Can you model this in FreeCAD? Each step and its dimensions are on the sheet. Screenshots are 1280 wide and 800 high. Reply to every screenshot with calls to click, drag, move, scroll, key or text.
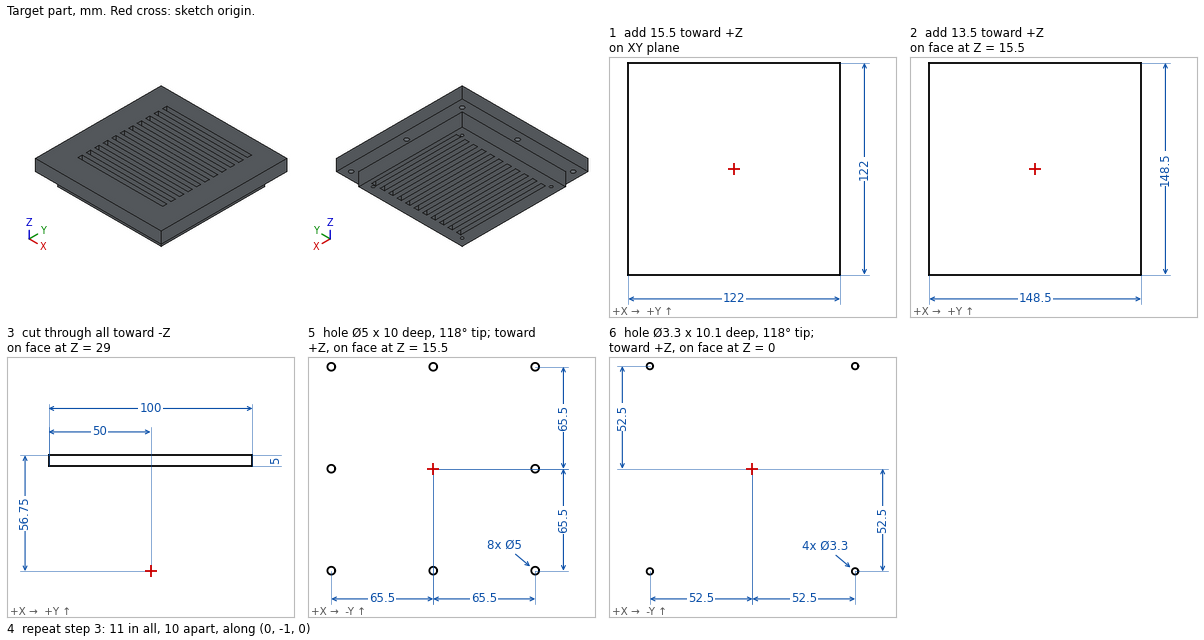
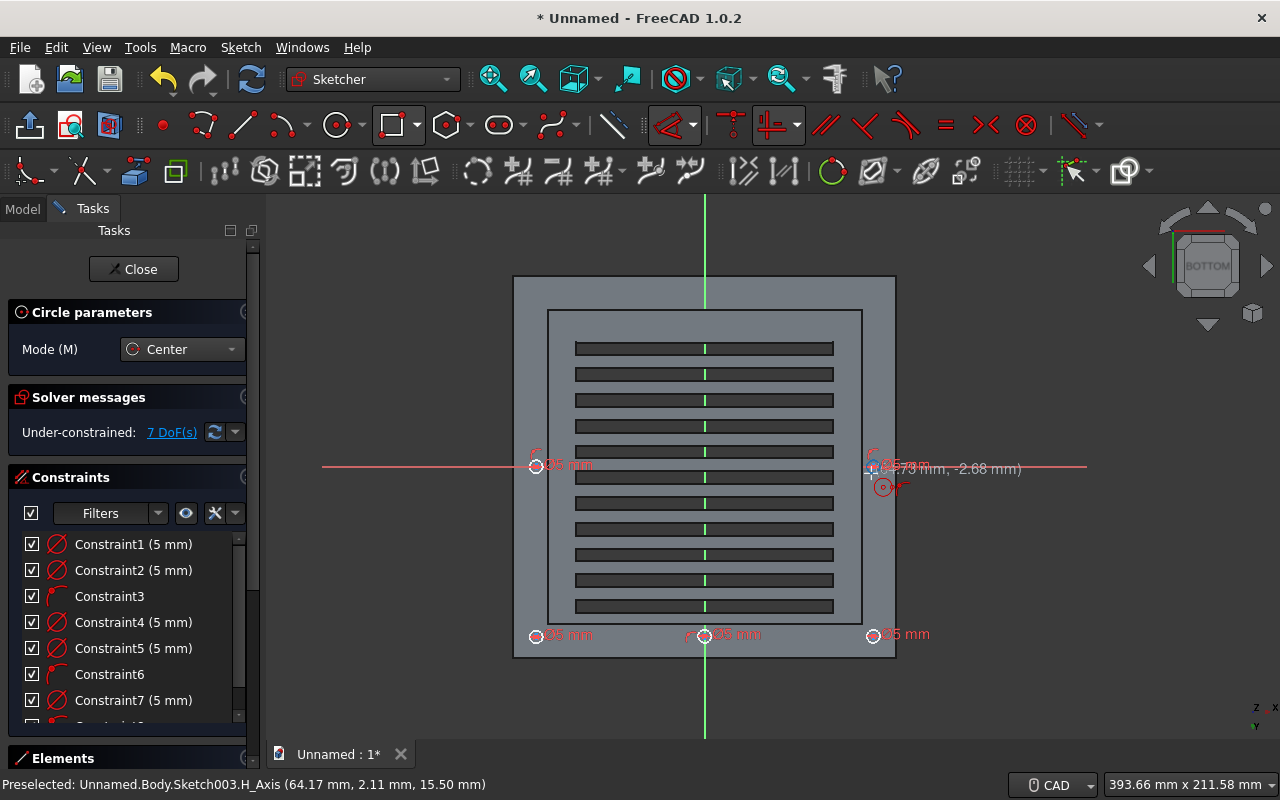
scroll(873, 298, up, 7)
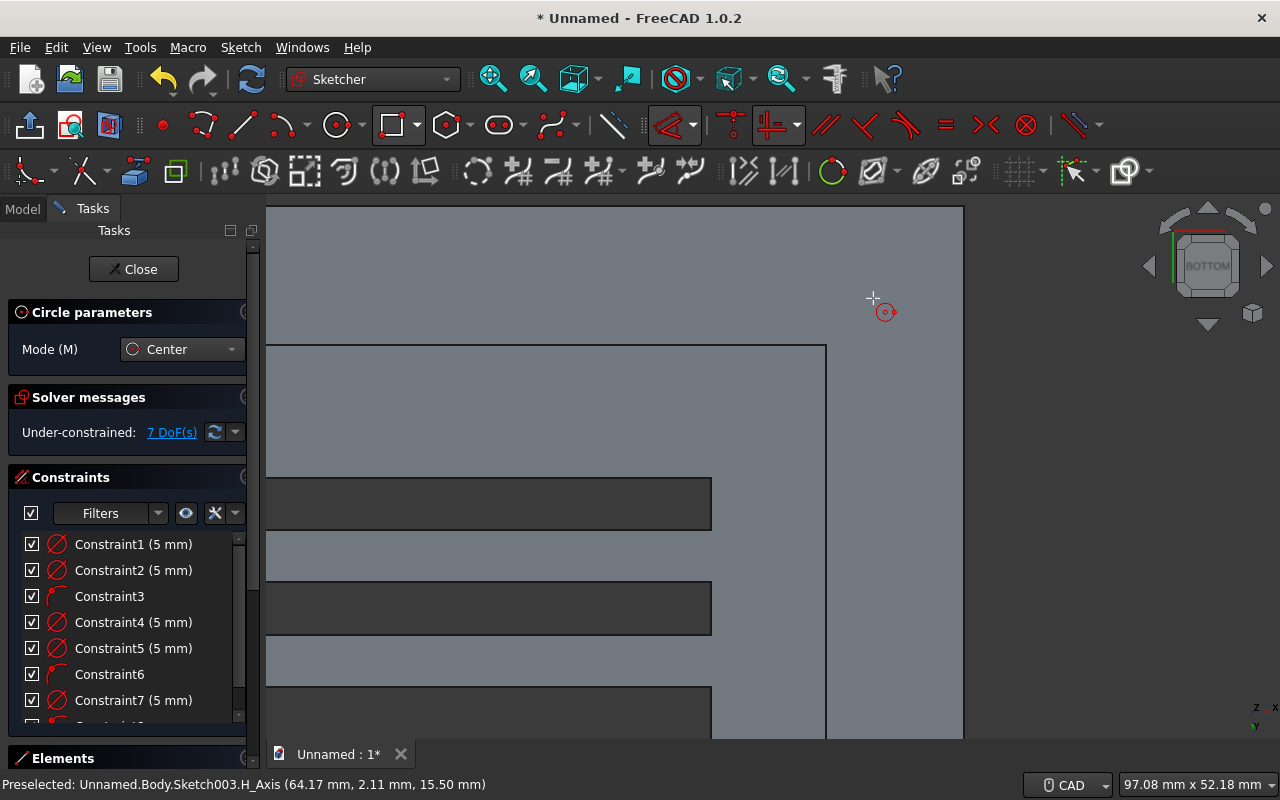
scroll(873, 298, down, 7)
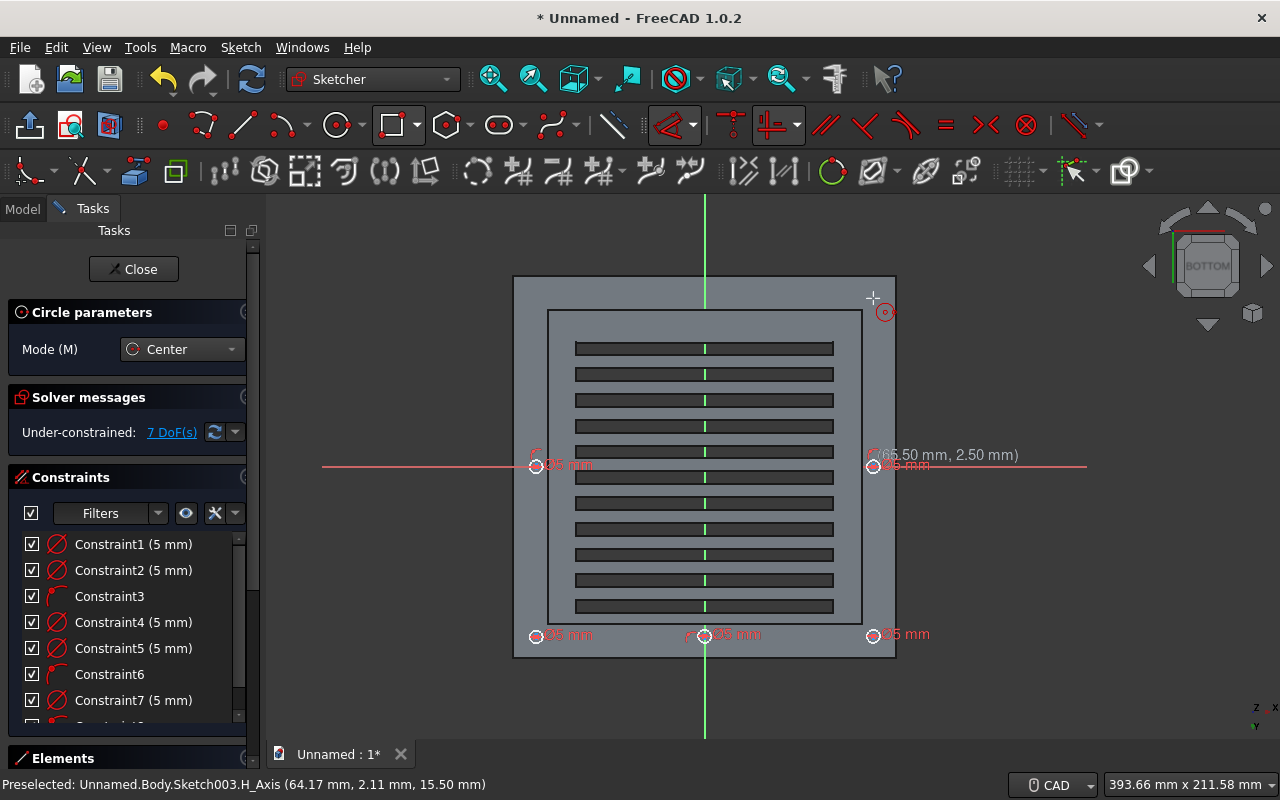
click(873, 298)
move(878, 294)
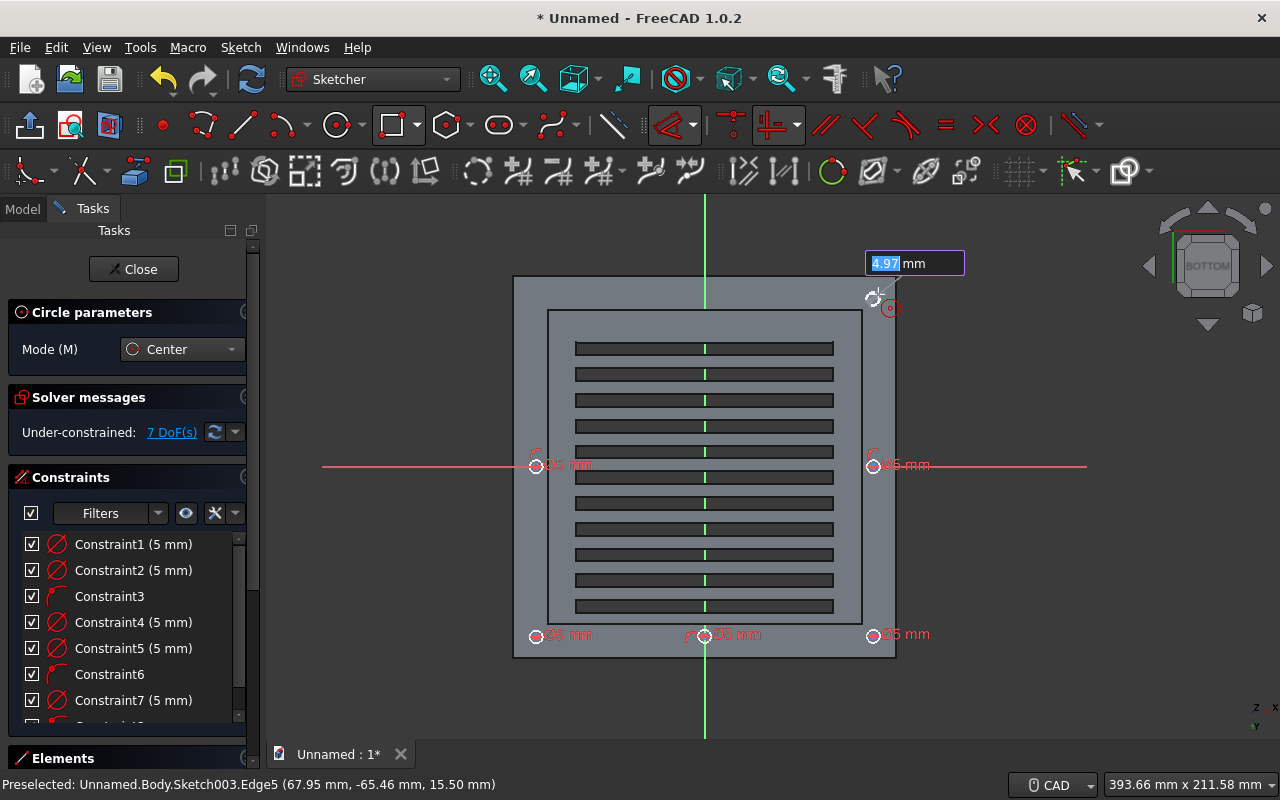
text(5)
key(Return)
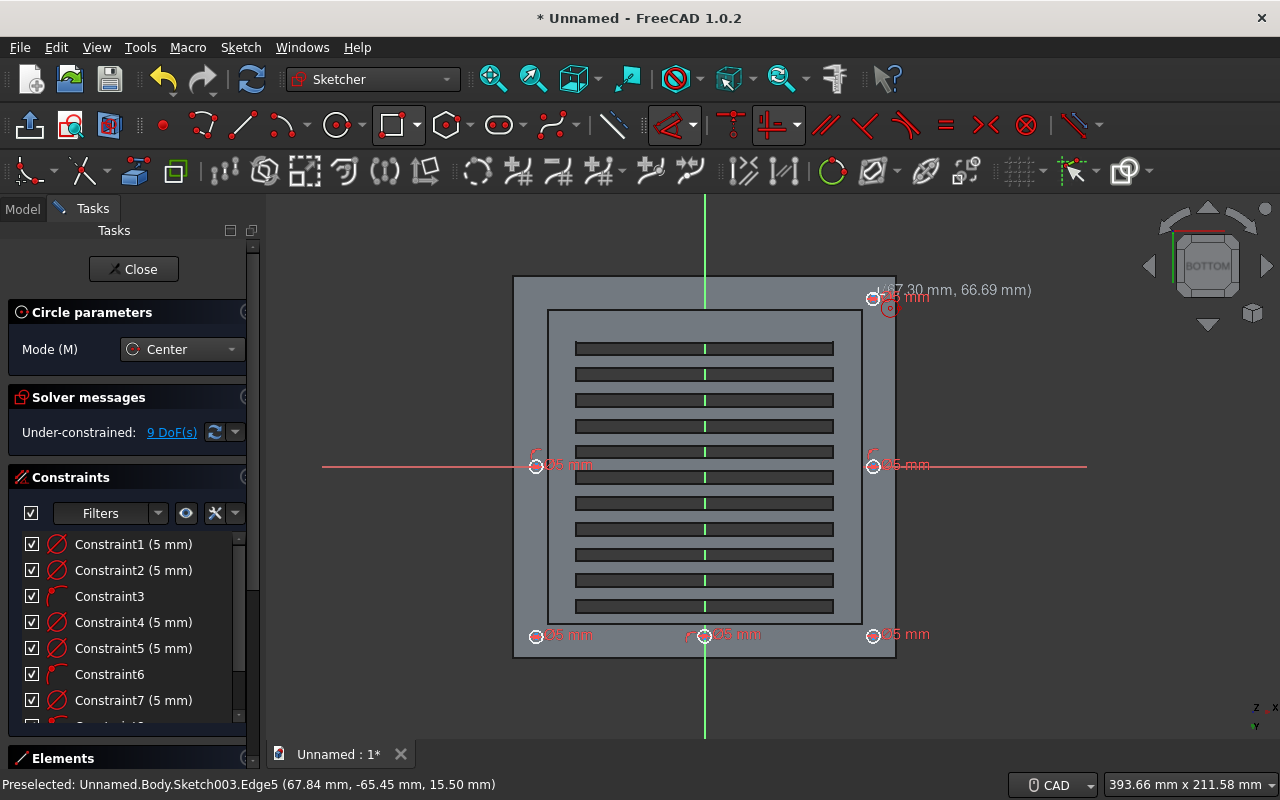
scroll(705, 298, up, 7)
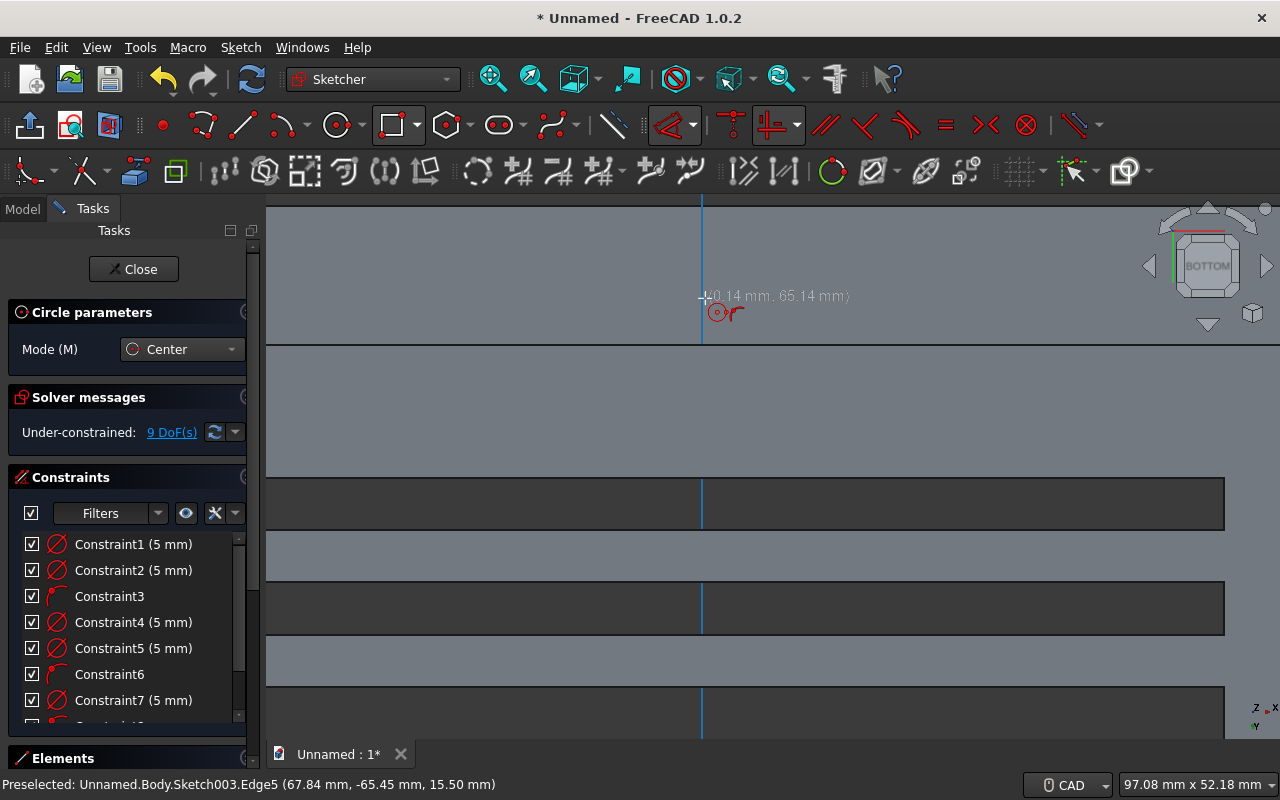
scroll(705, 298, down, 7)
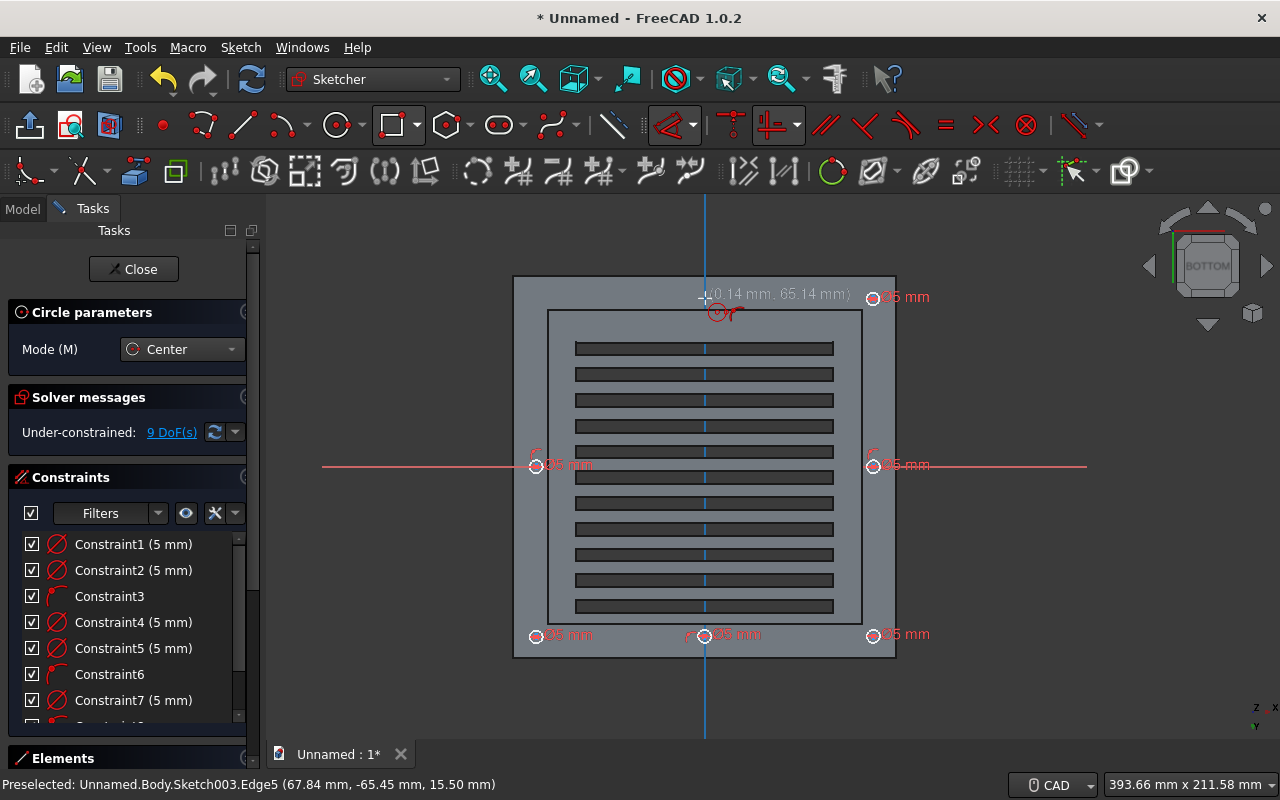
click(705, 298)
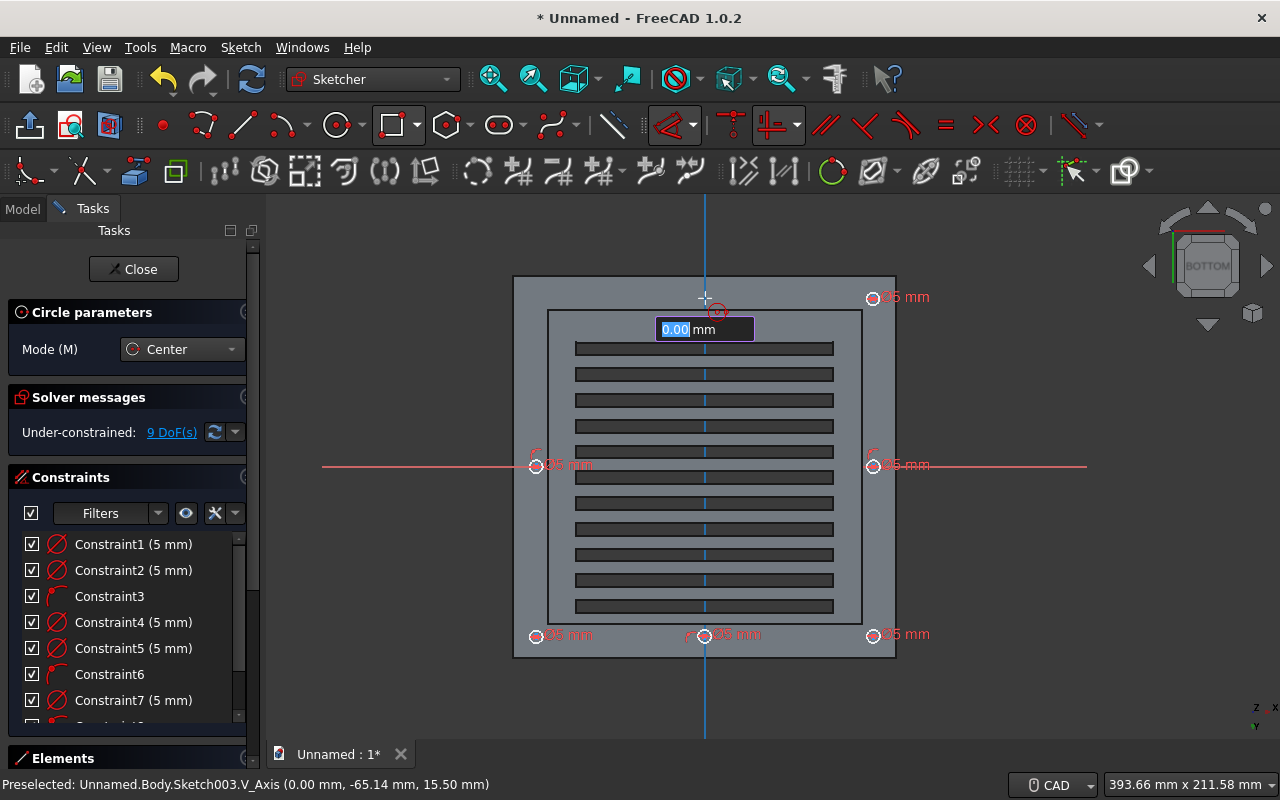
scroll(711, 296, up, 5)
move(709, 295)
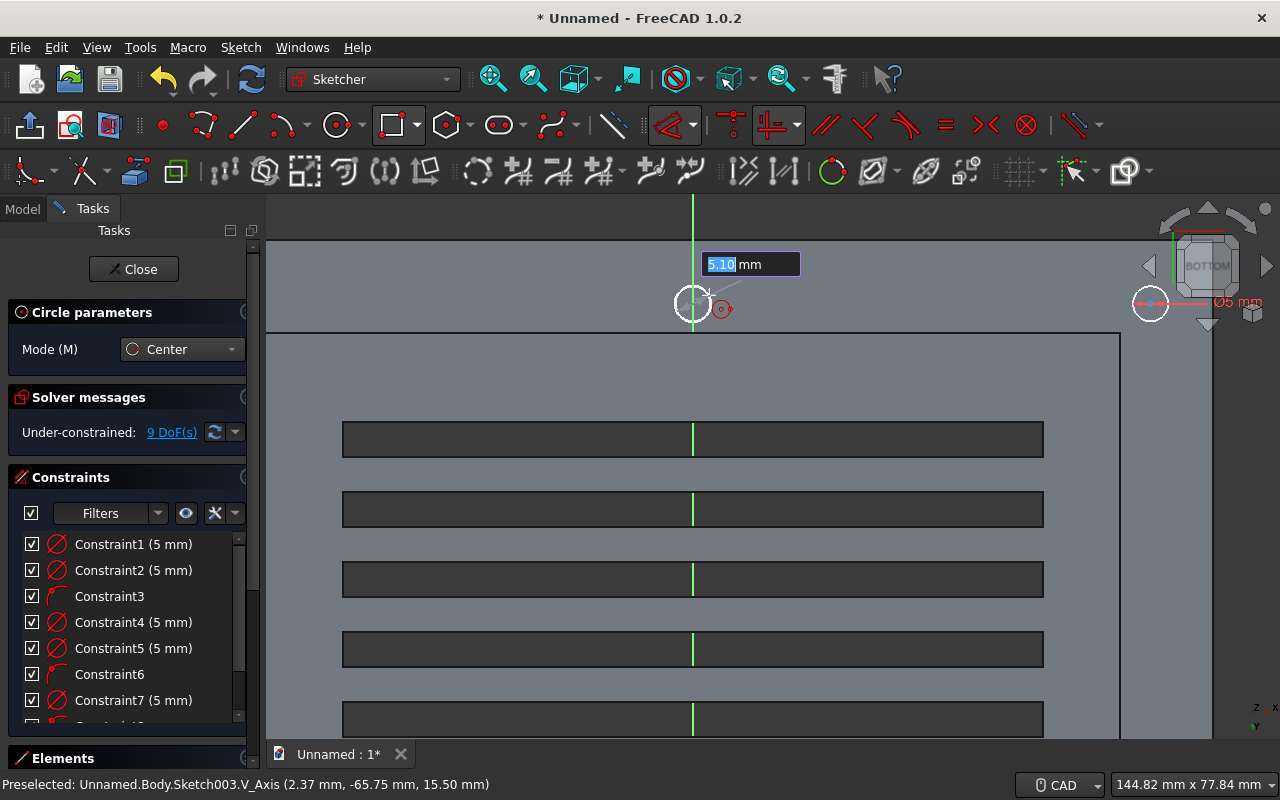
text(5)
key(Return)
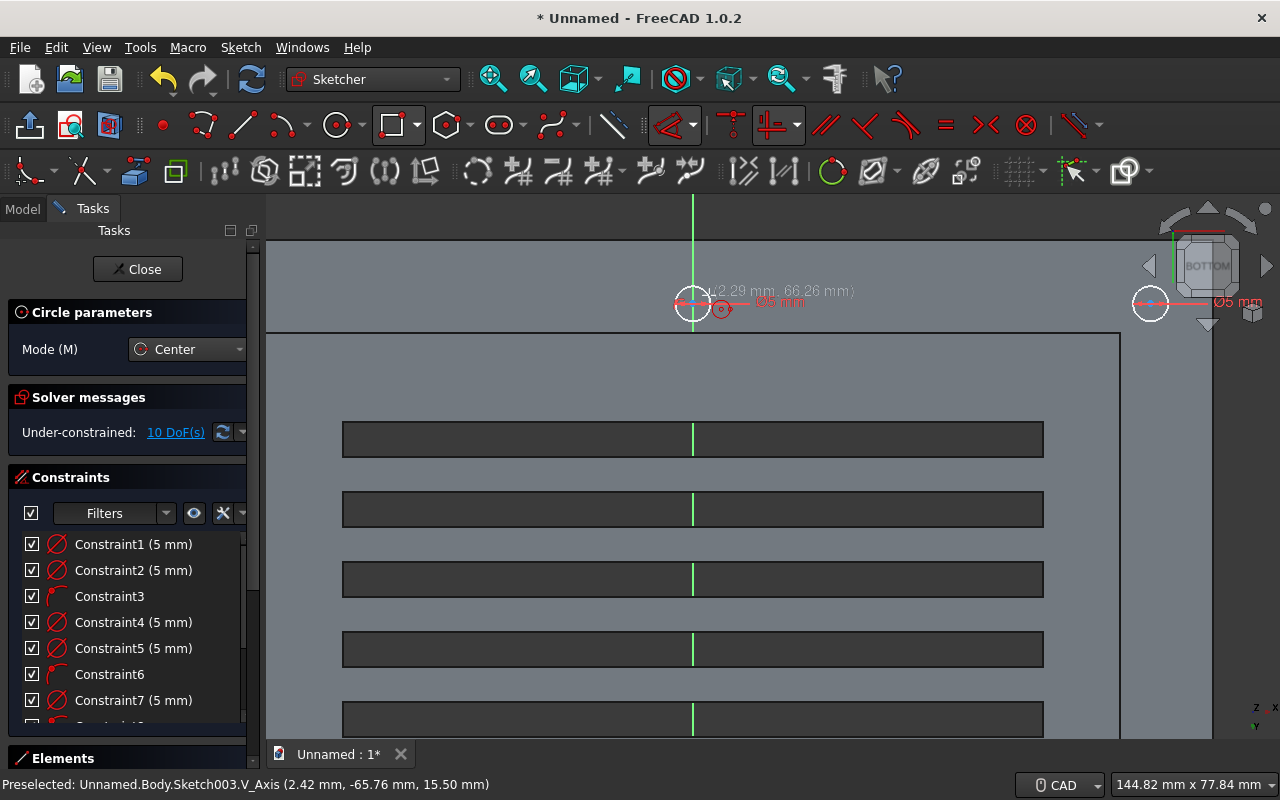
scroll(711, 296, down, 5)